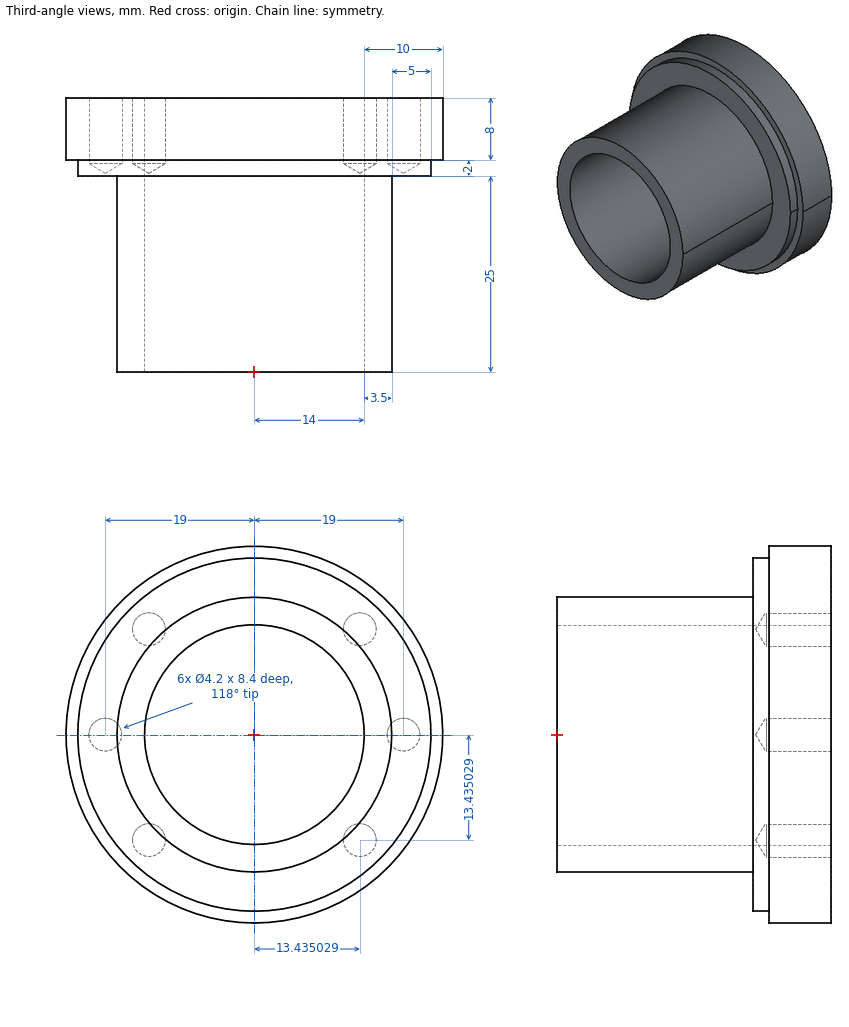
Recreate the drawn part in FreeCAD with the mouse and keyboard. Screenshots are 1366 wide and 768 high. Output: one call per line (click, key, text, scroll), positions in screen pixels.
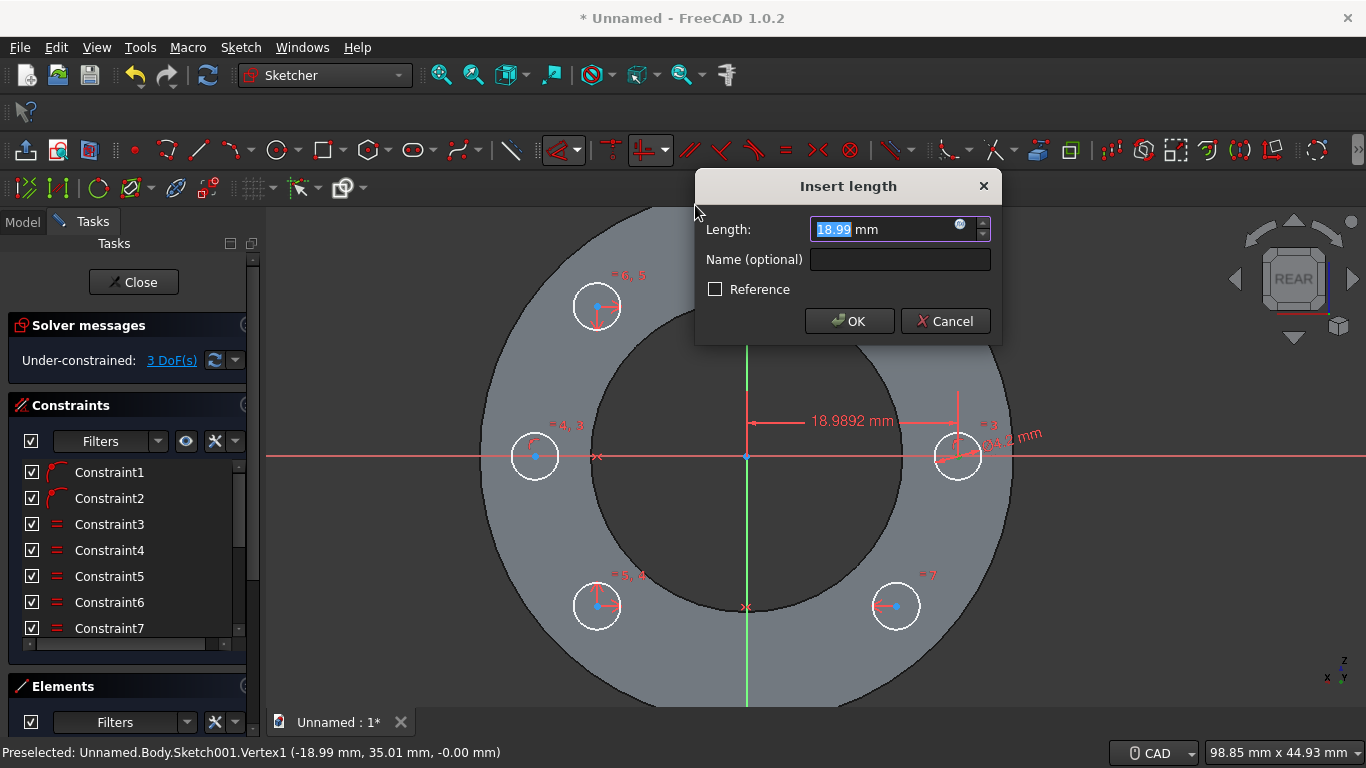
text(19)
key(Return)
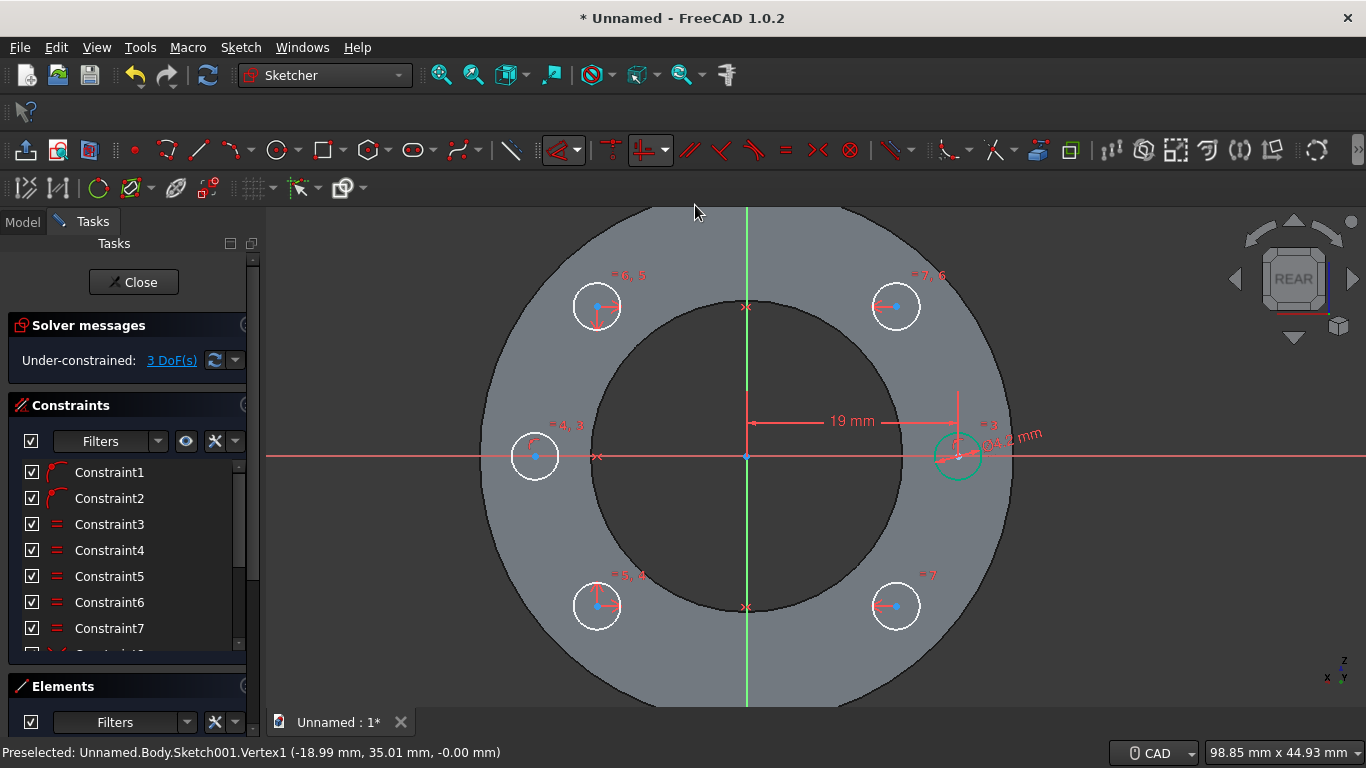
click(535, 456)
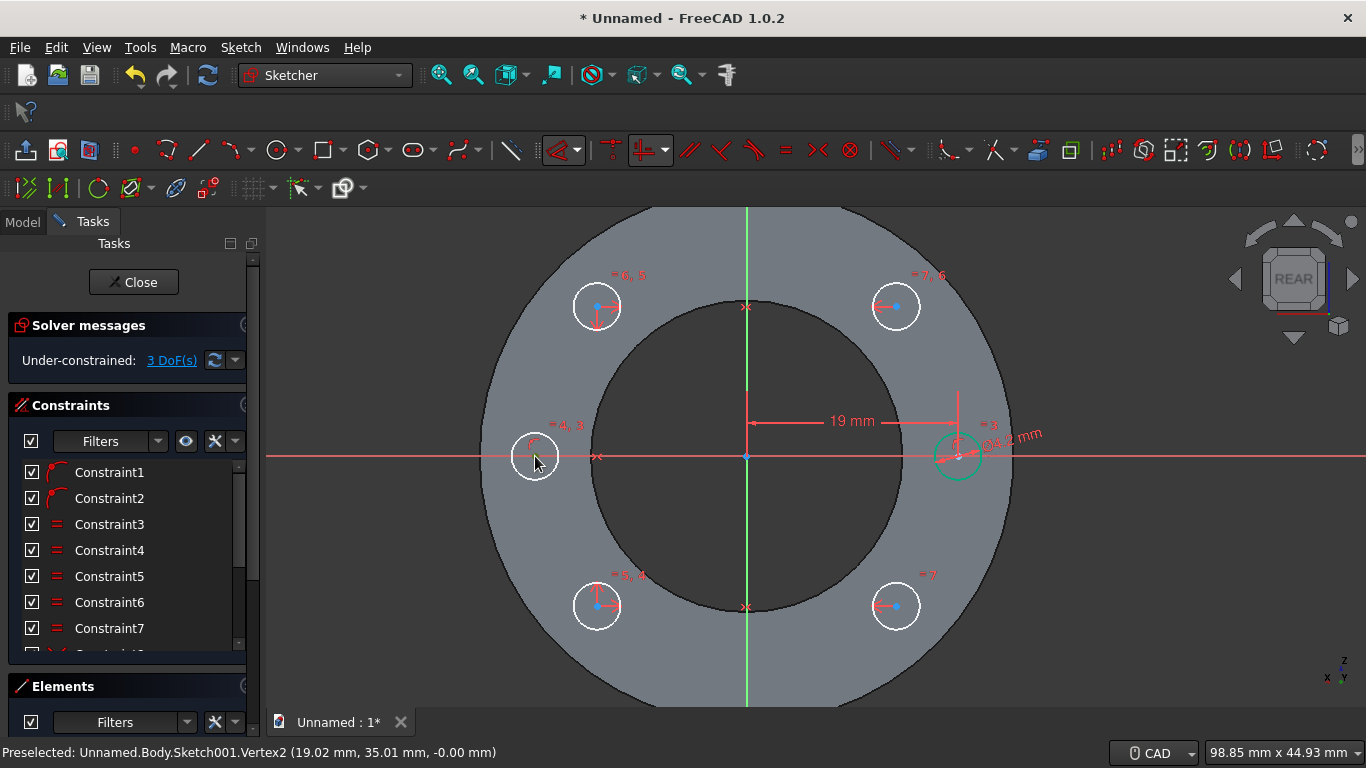
click(580, 150)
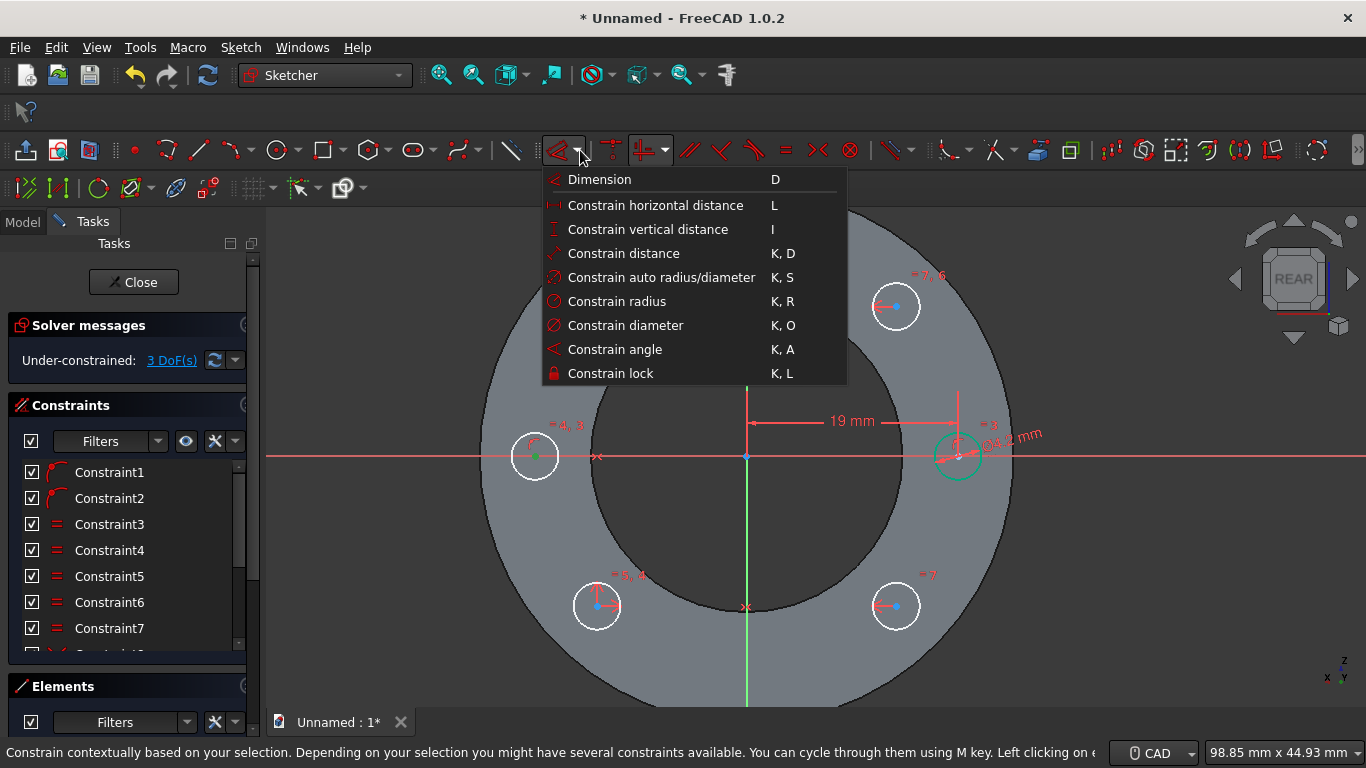
click(695, 205)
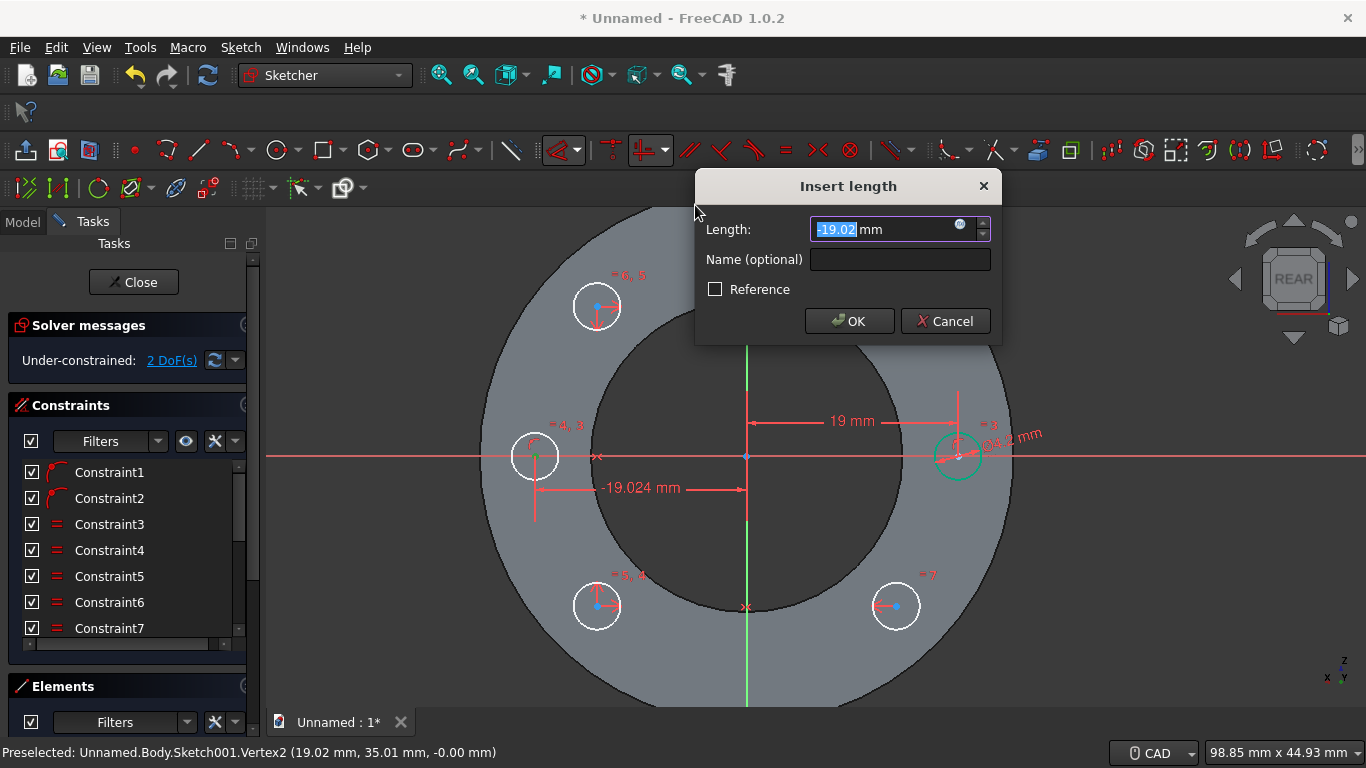
text(-19)
key(Return)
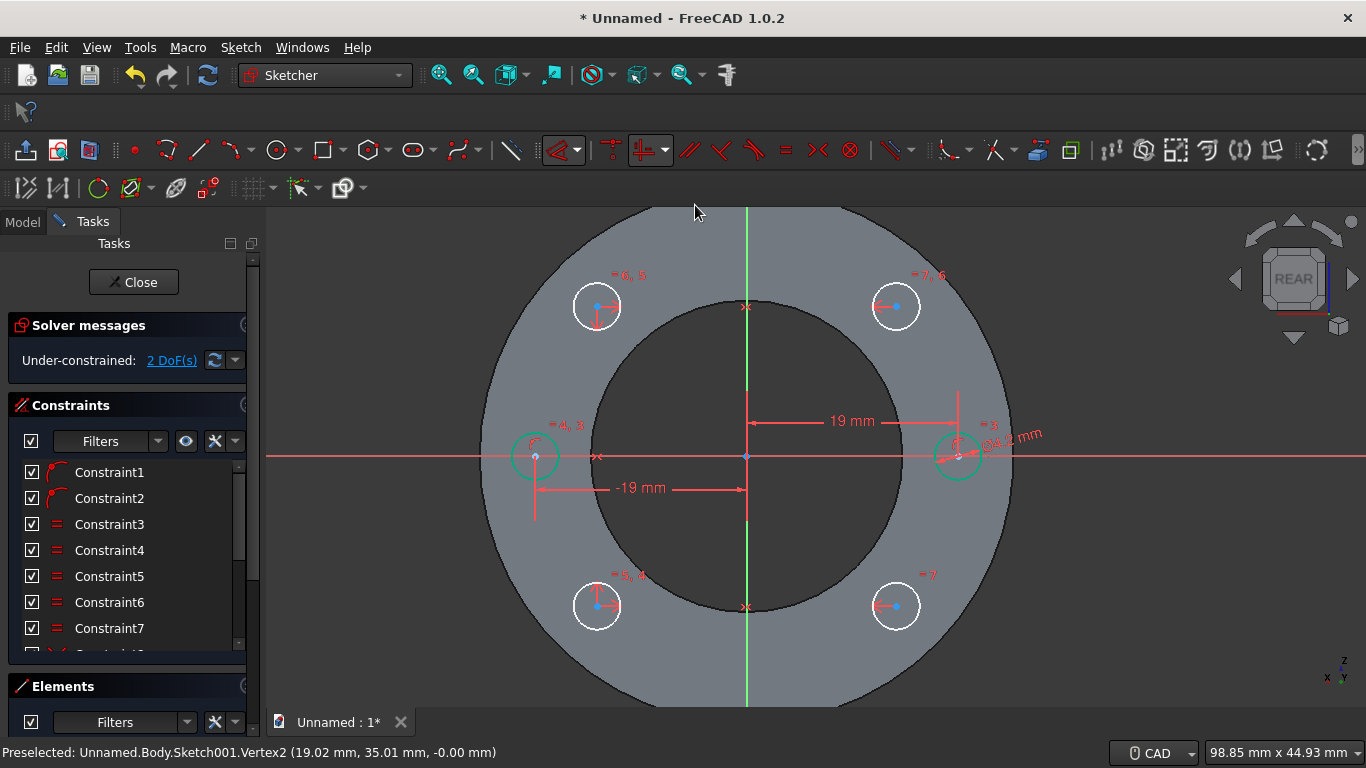
click(597, 606)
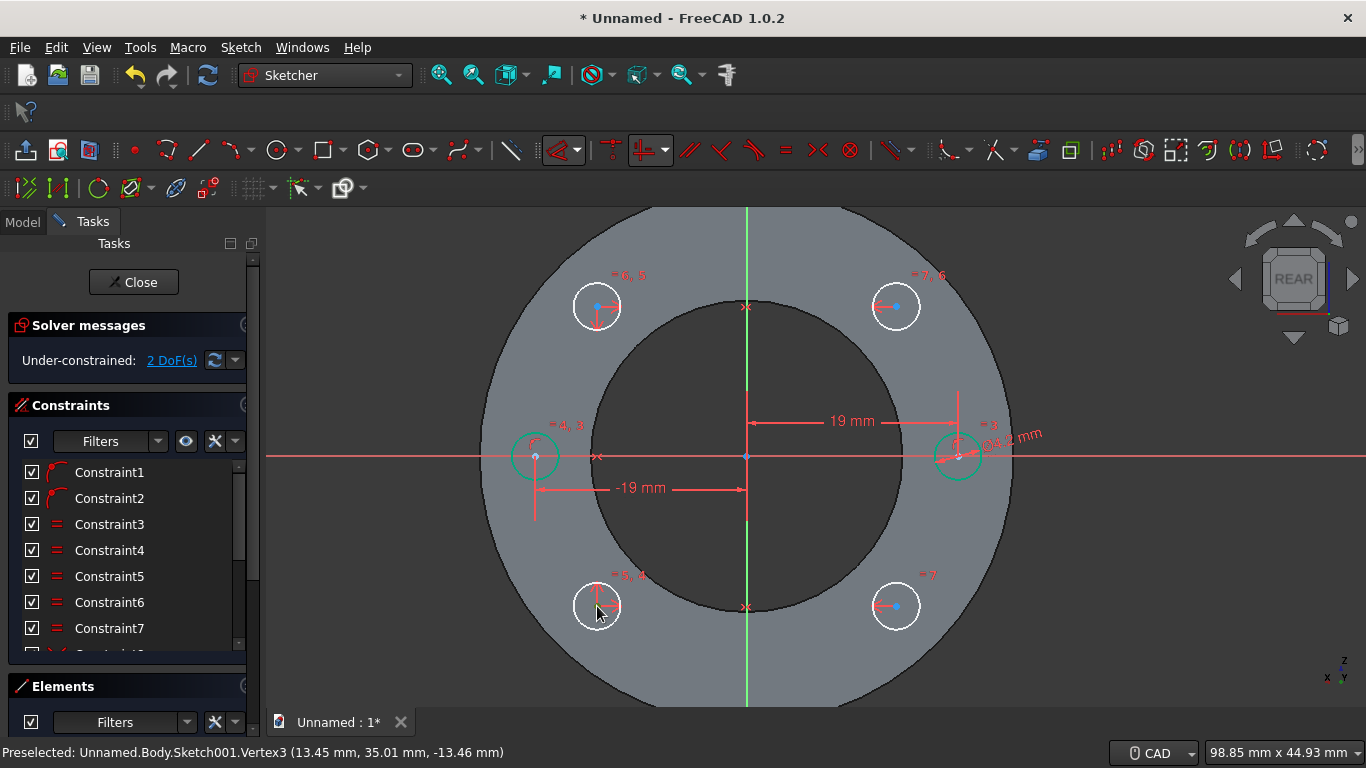
key(l)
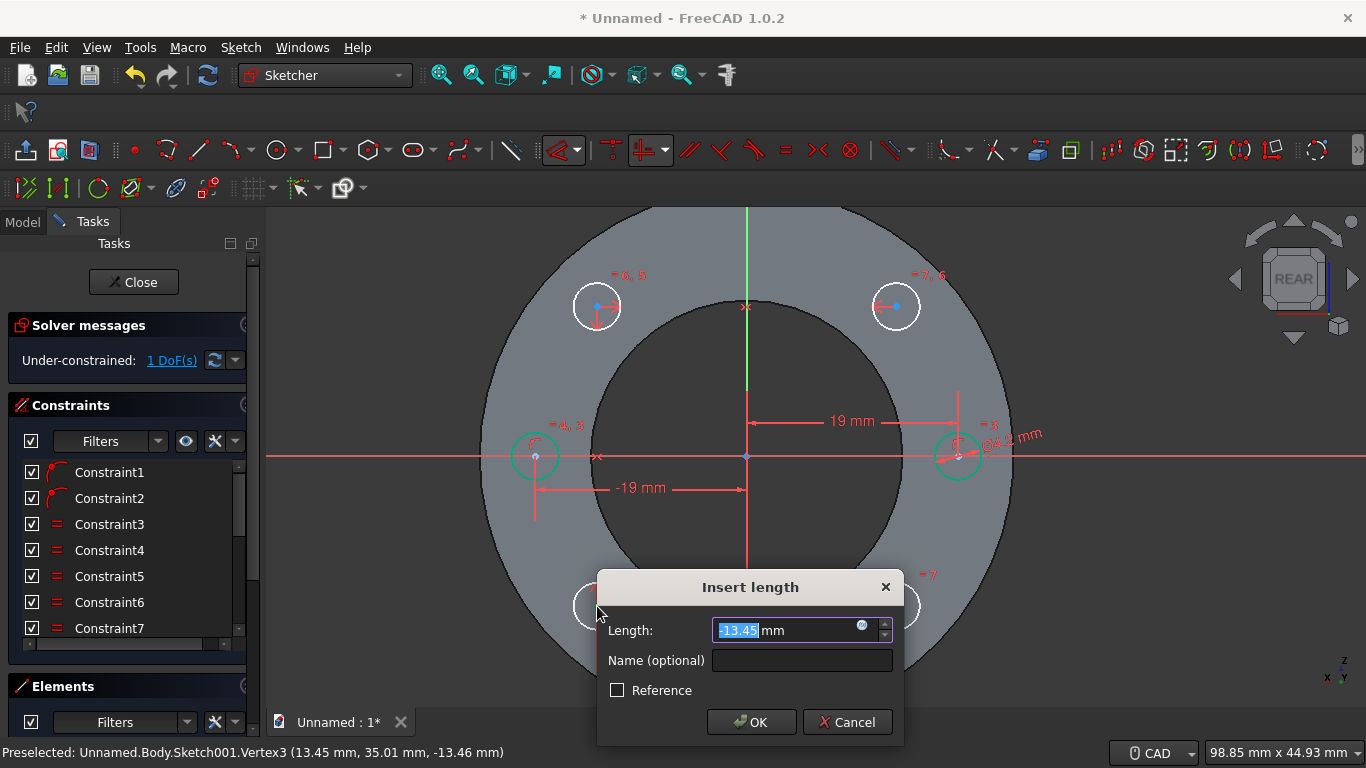
text(-13.435029)
key(Return)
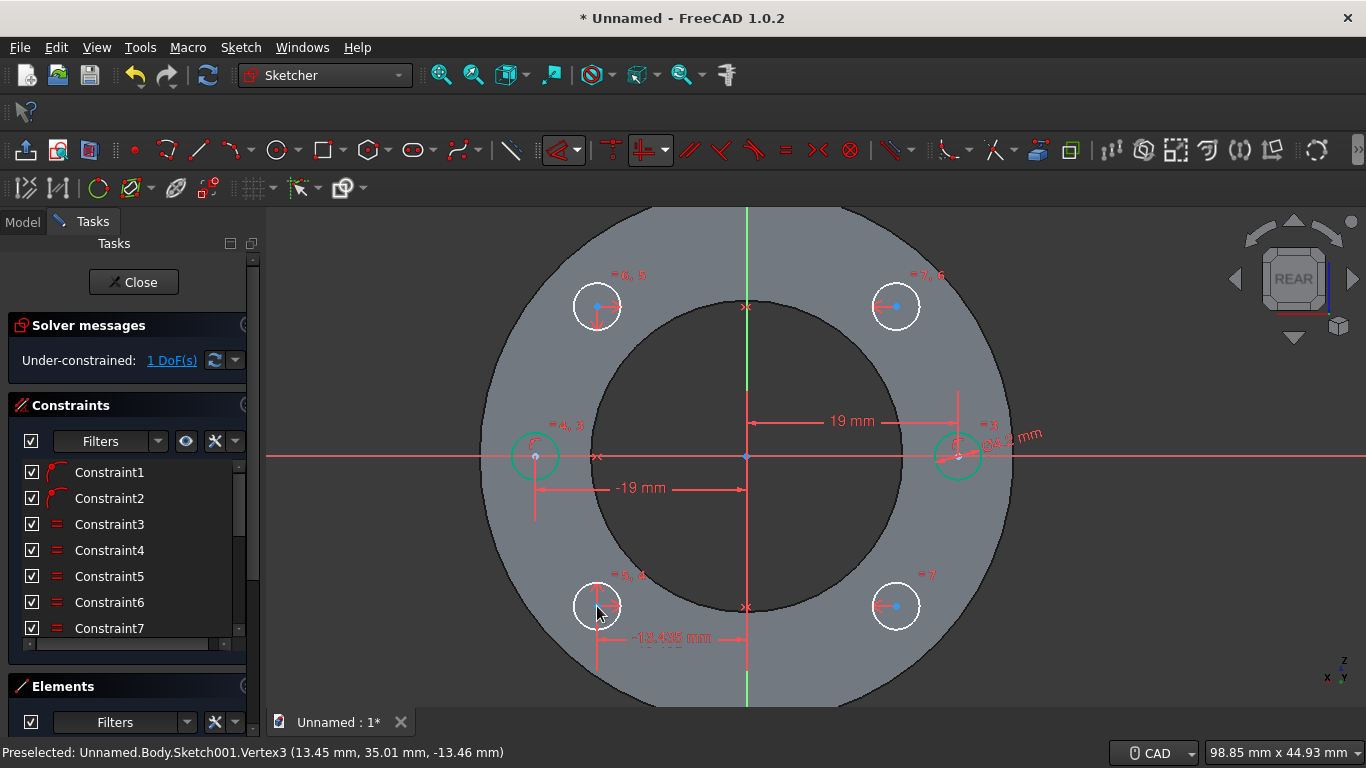
click(597, 606)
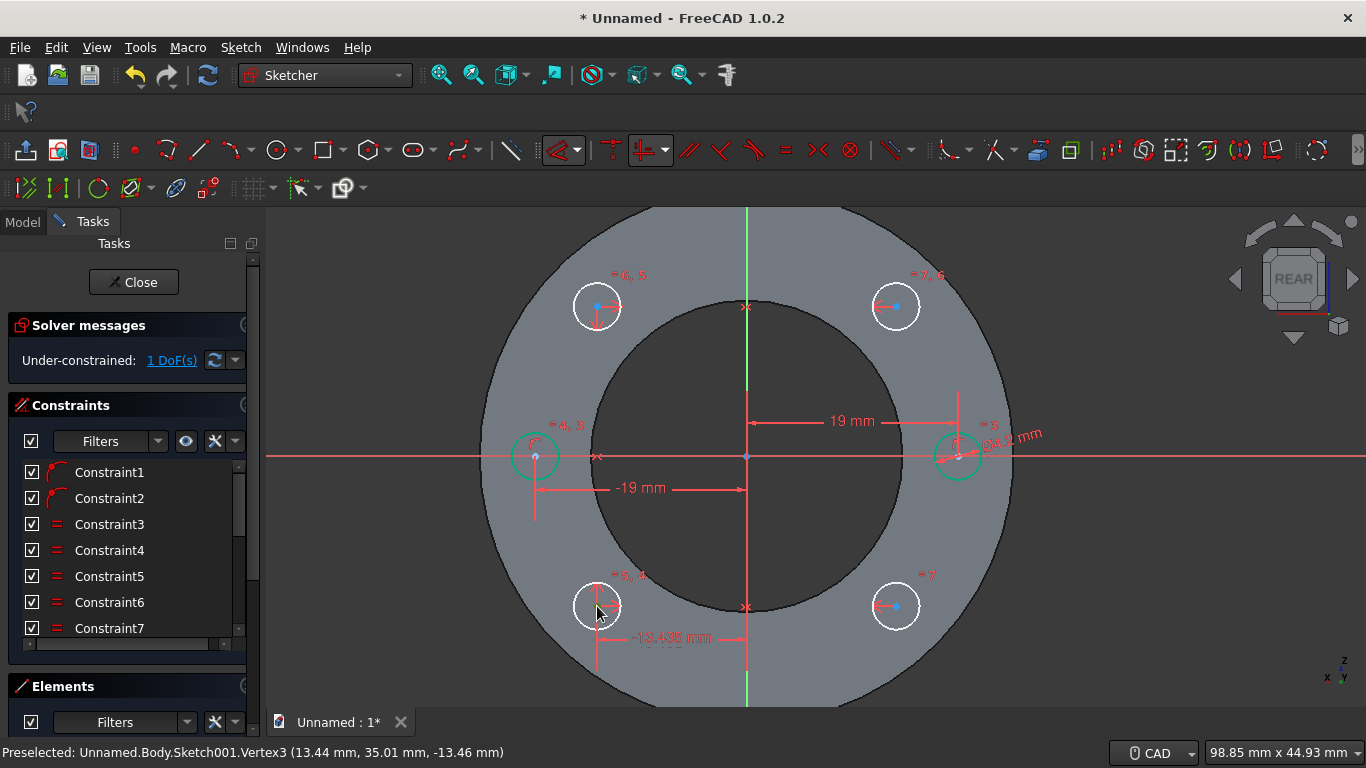
key(i)